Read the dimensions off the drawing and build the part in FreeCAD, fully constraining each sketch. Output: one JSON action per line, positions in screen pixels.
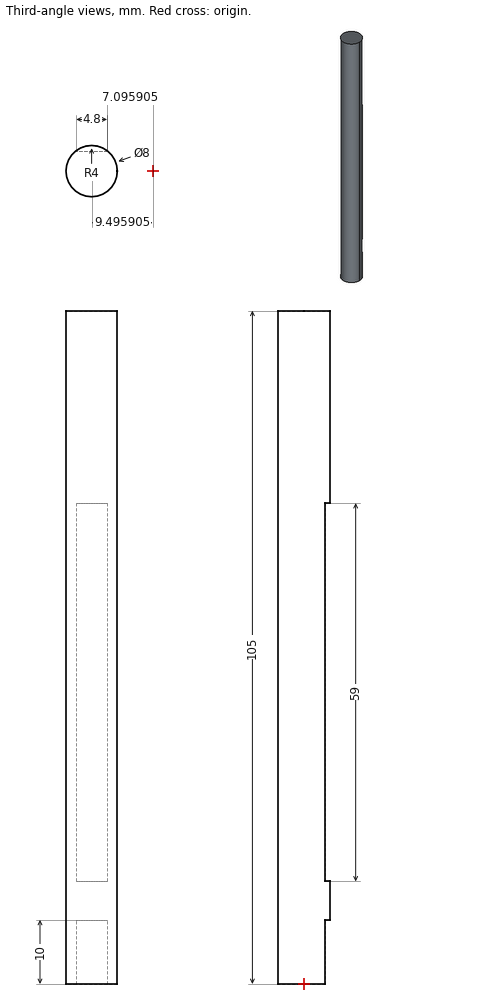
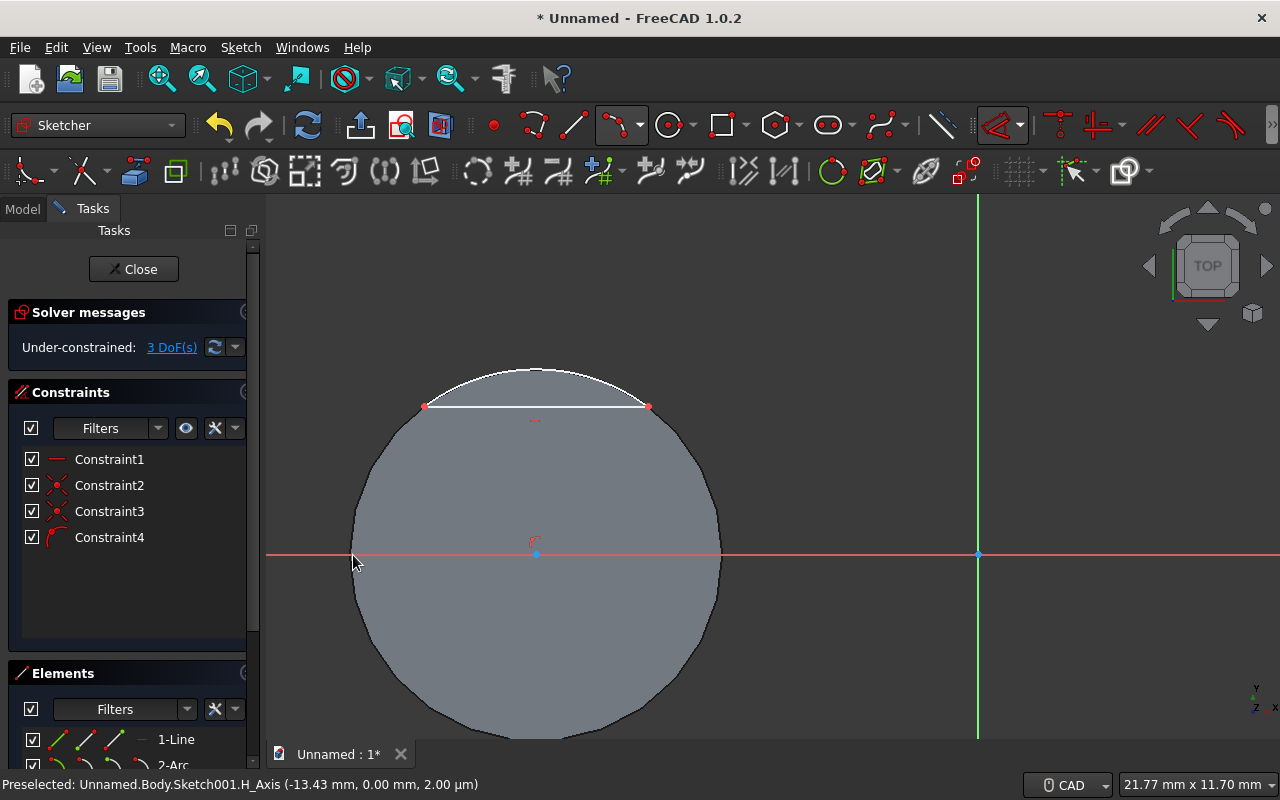
{"action": "left_click", "coordinate": [584, 376]}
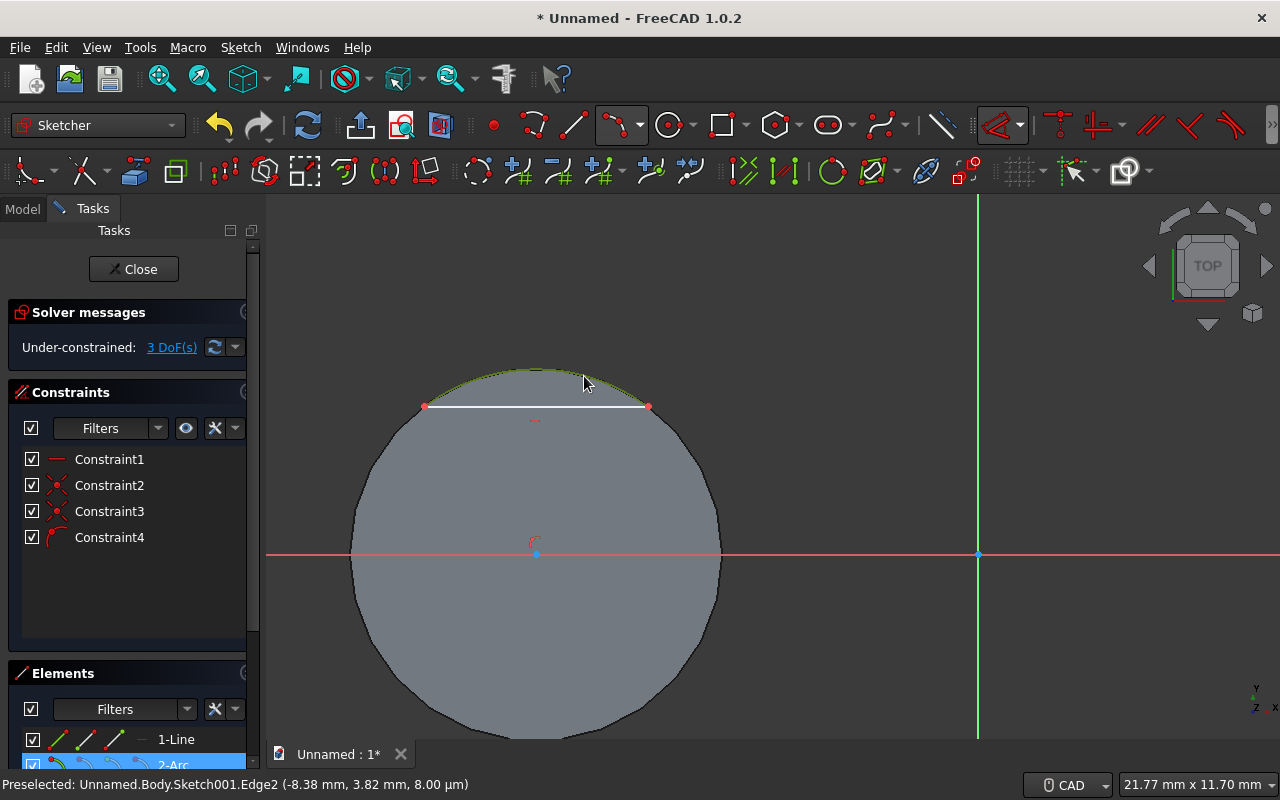
{"action": "key", "text": "k r"}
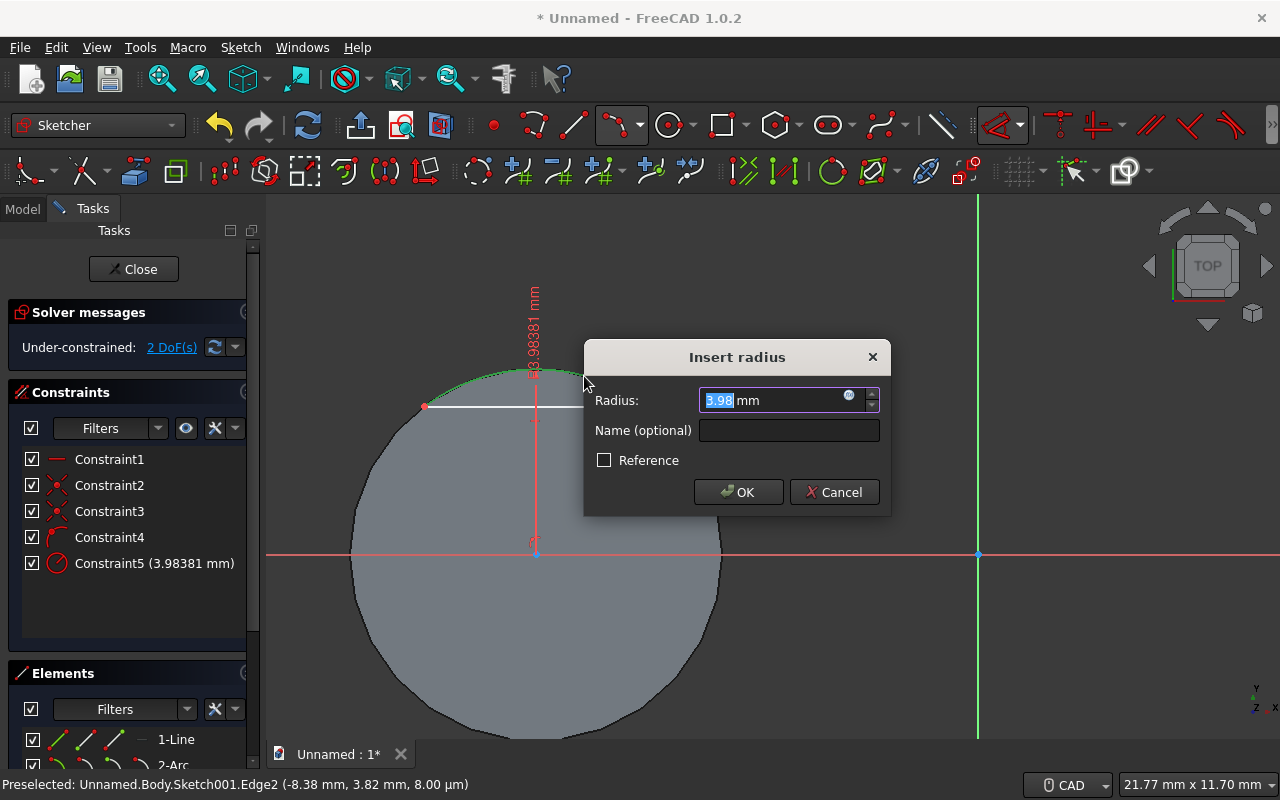
{"action": "type", "text": "4"}
{"action": "key", "text": "Return"}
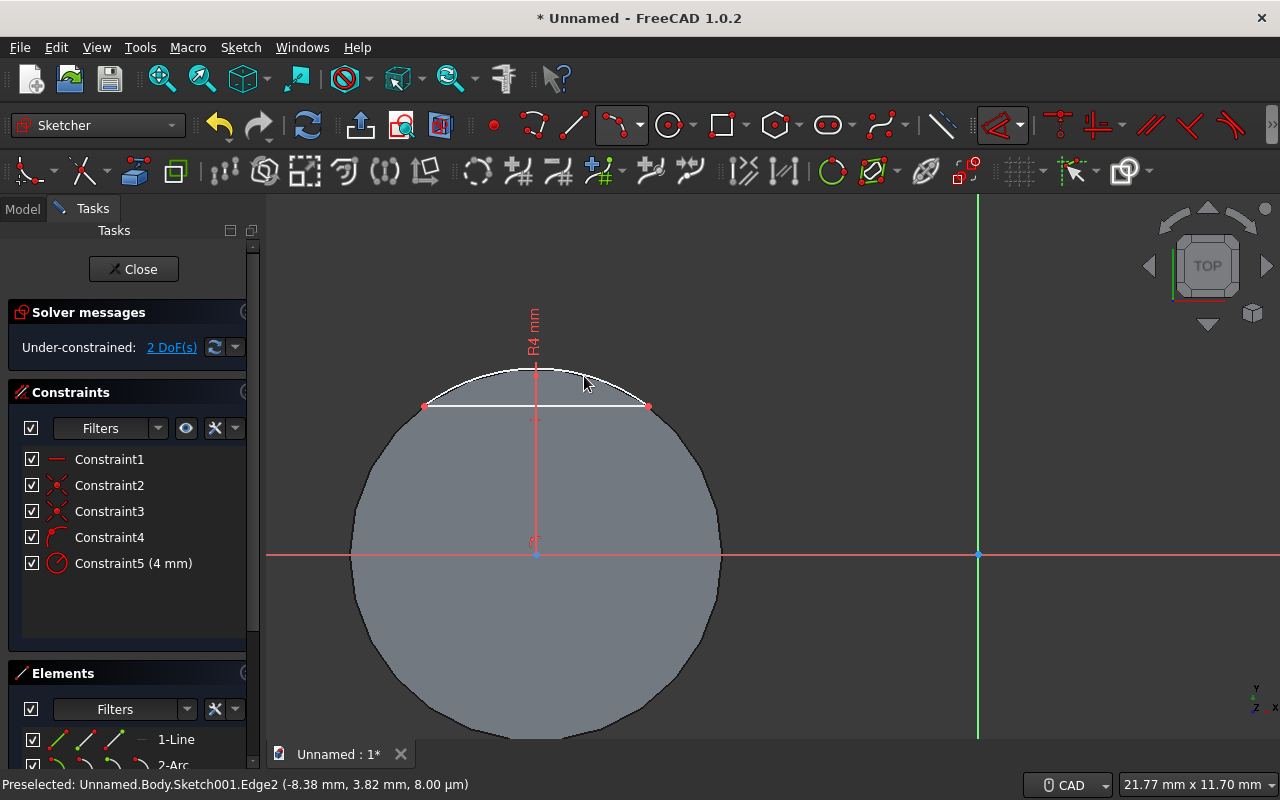
{"action": "left_click", "coordinate": [581, 406]}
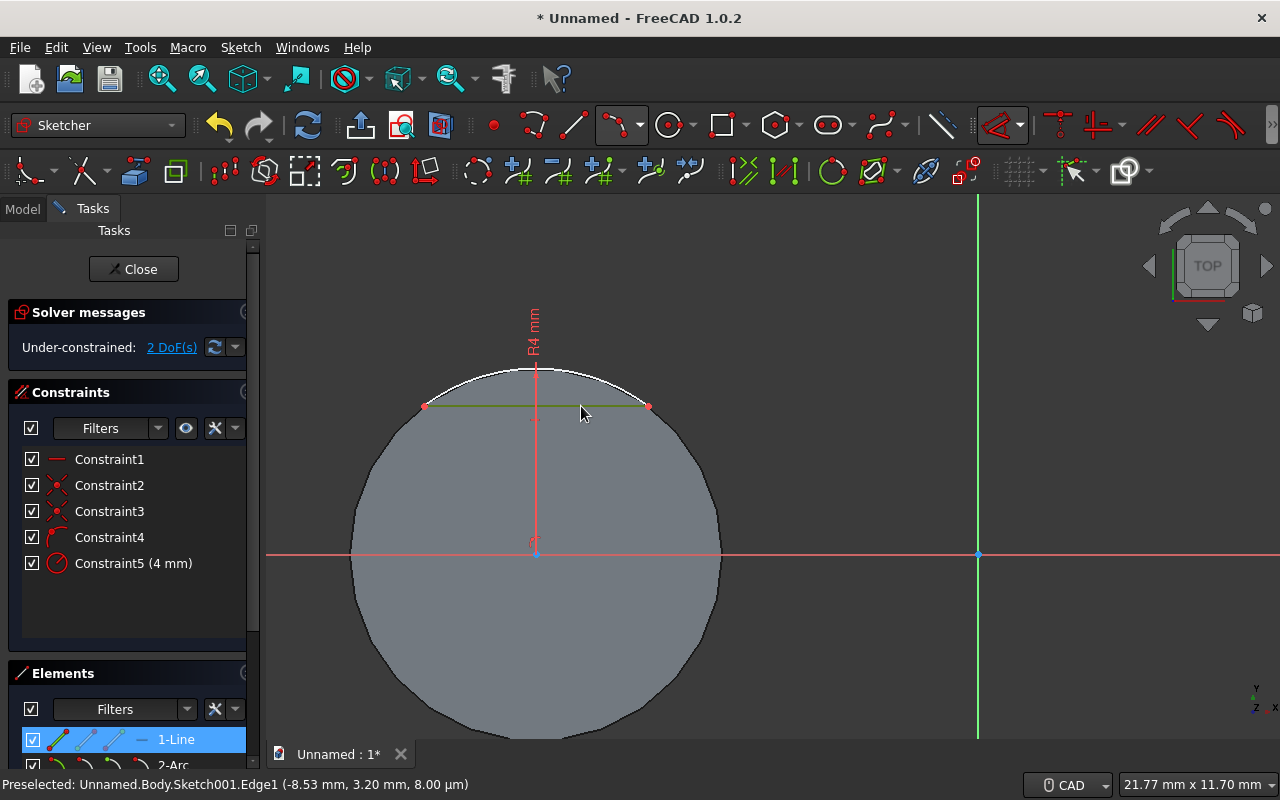
{"action": "key", "text": "l"}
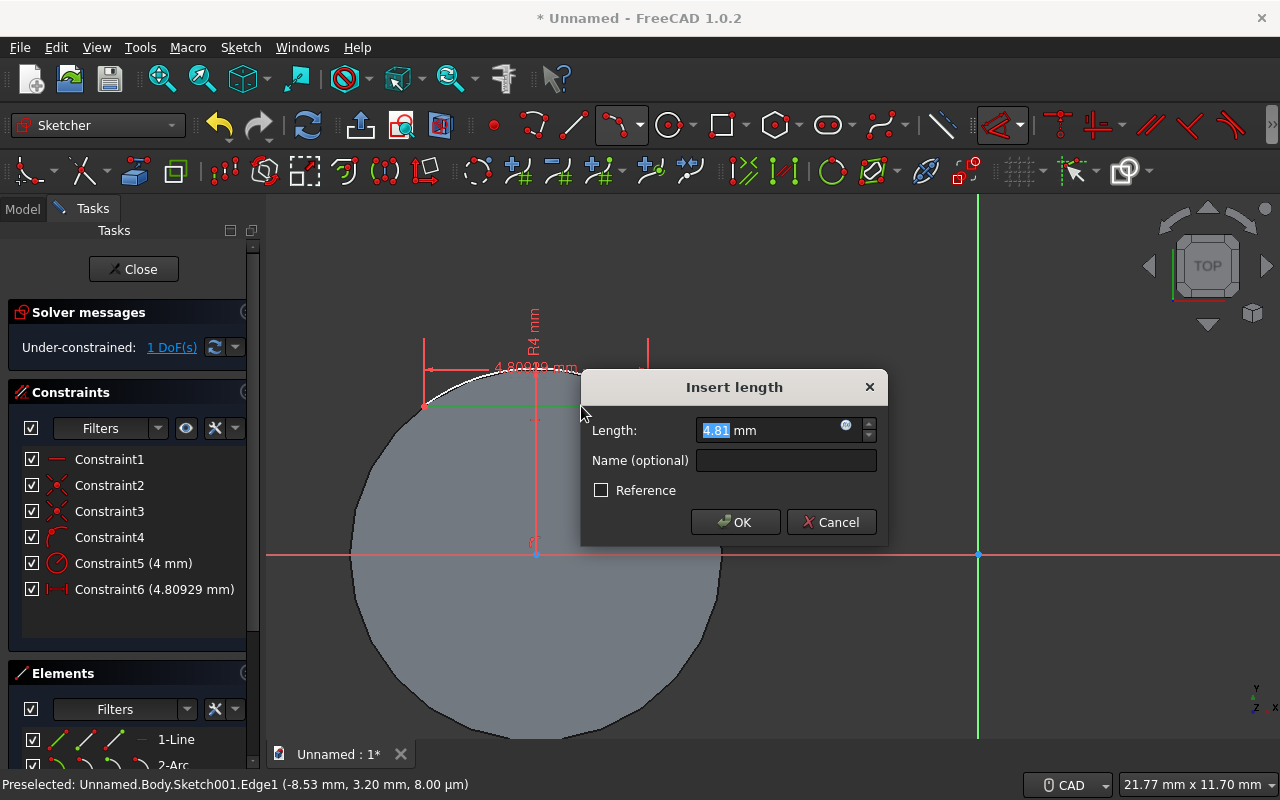
{"action": "type", "text": "4.8"}
{"action": "key", "text": "Return"}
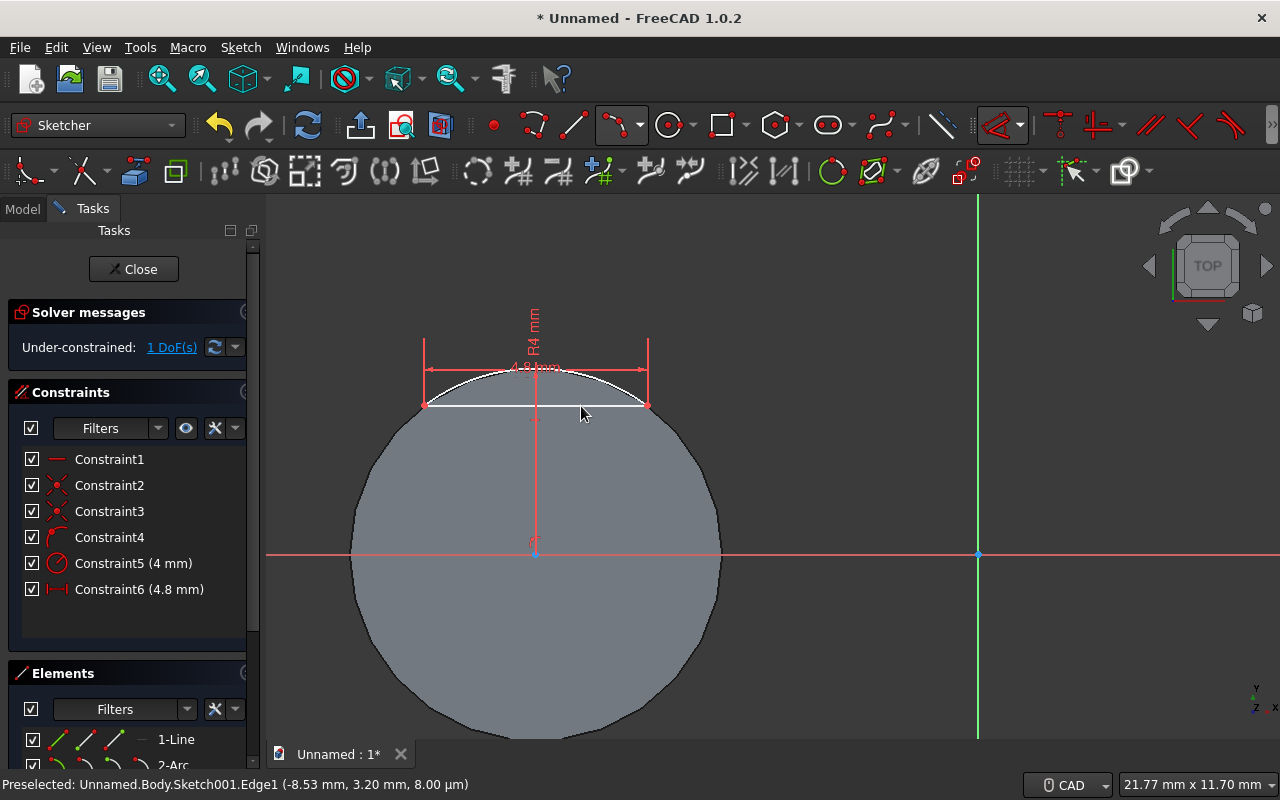
{"action": "left_click", "coordinate": [648, 406]}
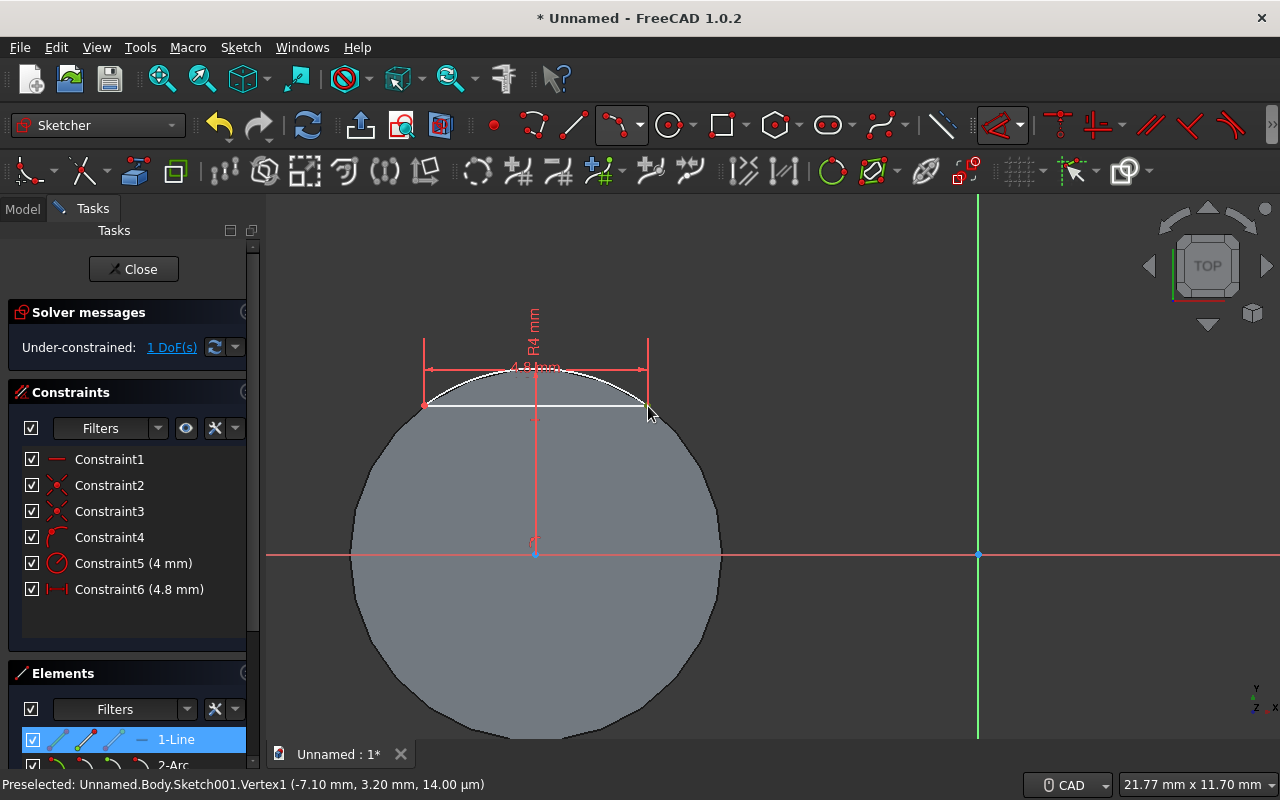
{"action": "key", "text": "l"}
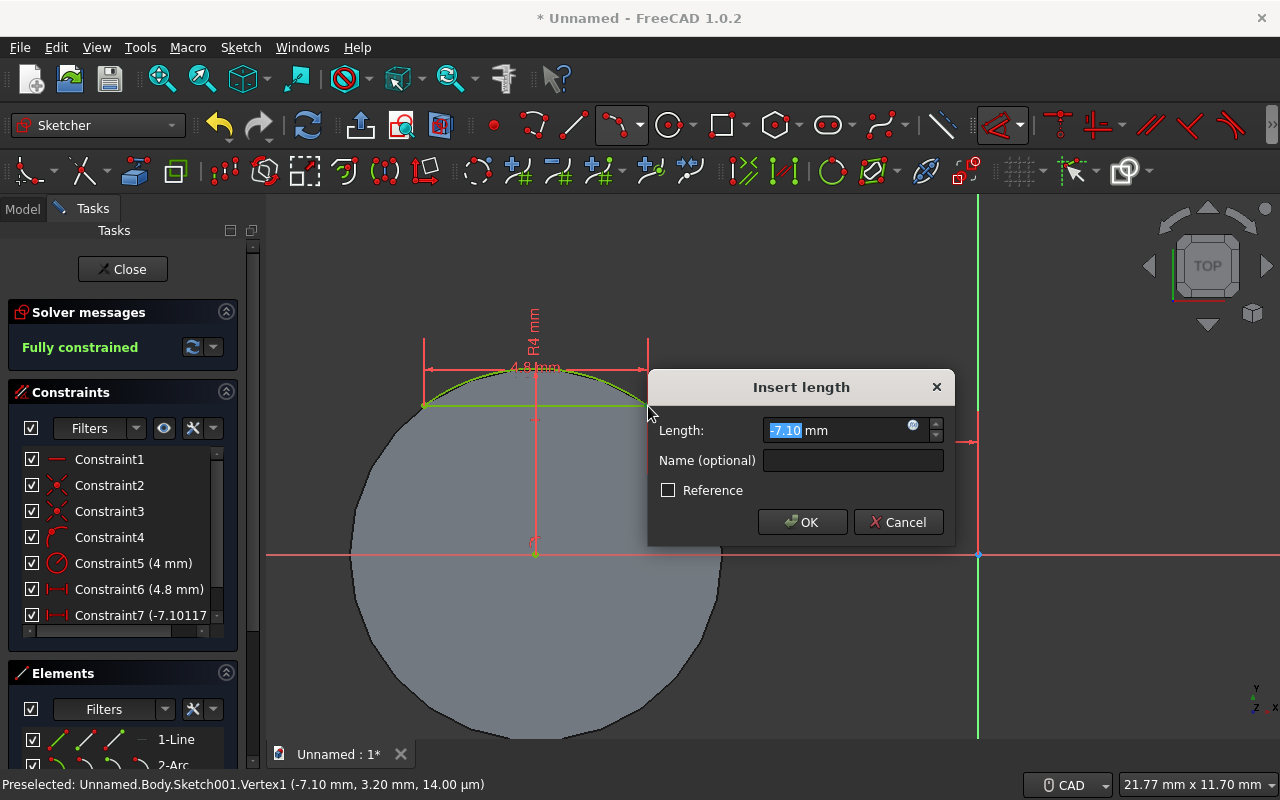
{"action": "type", "text": "-7.095905"}
{"action": "key", "text": "Return"}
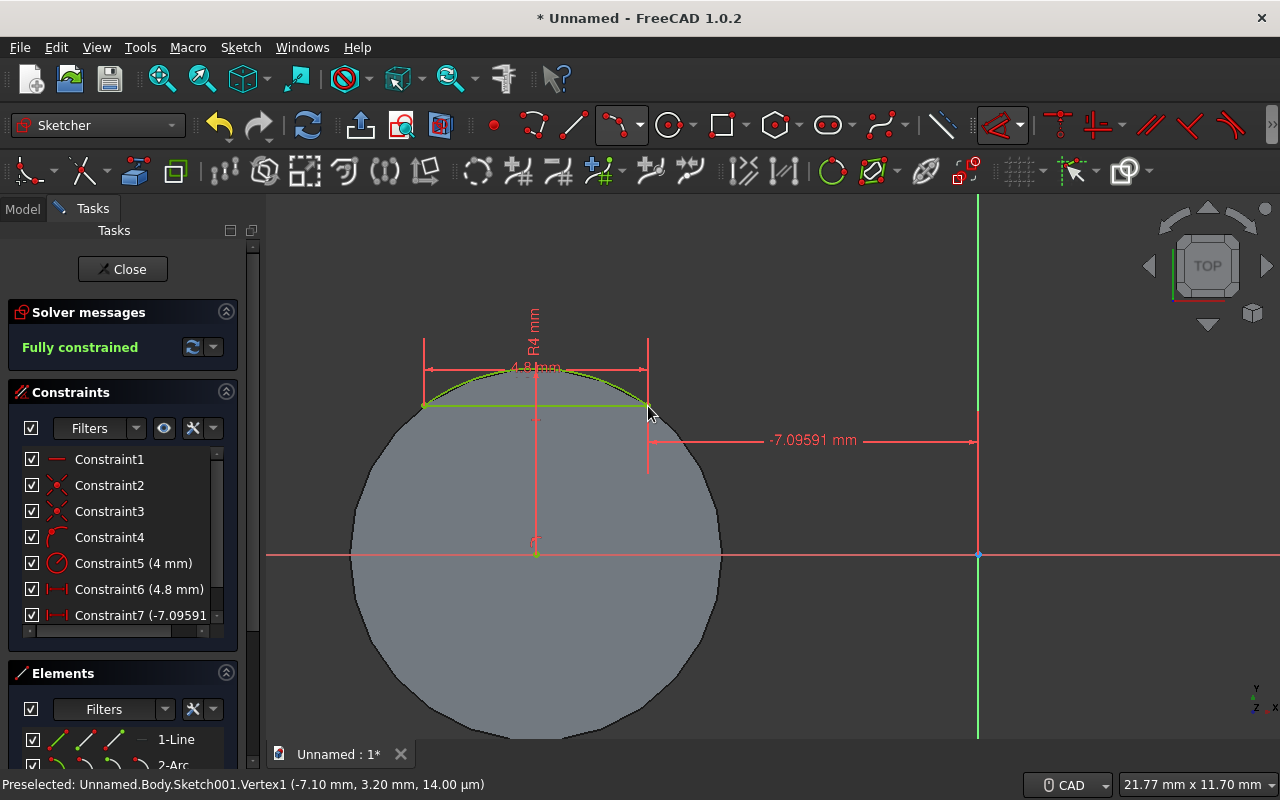
{"action": "left_click", "coordinate": [123, 269]}